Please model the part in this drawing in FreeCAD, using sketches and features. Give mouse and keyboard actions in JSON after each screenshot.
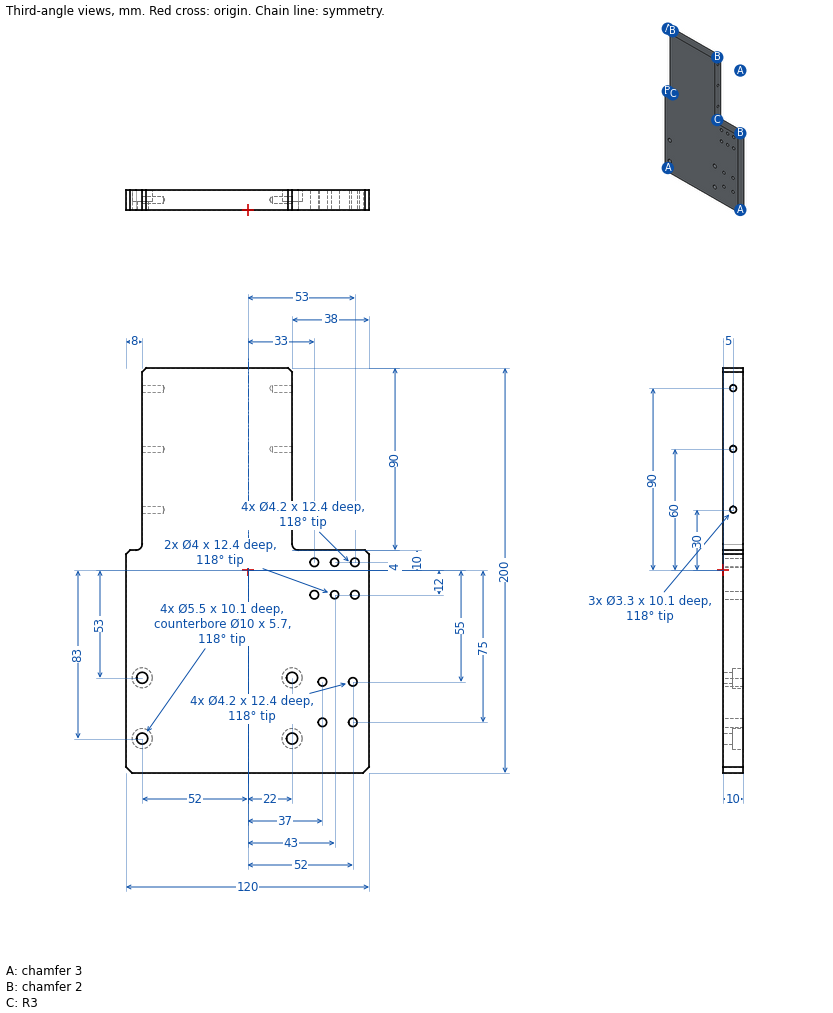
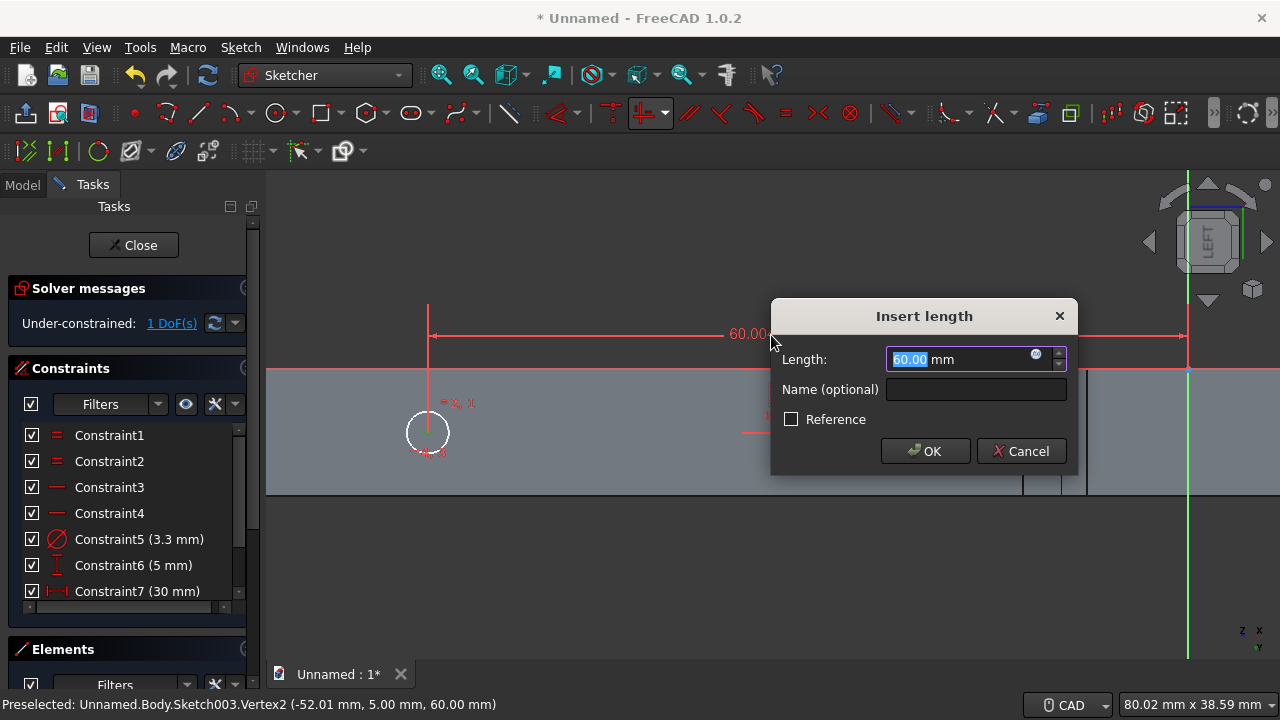
{"action": "type", "text": "60"}
{"action": "key", "text": "Return"}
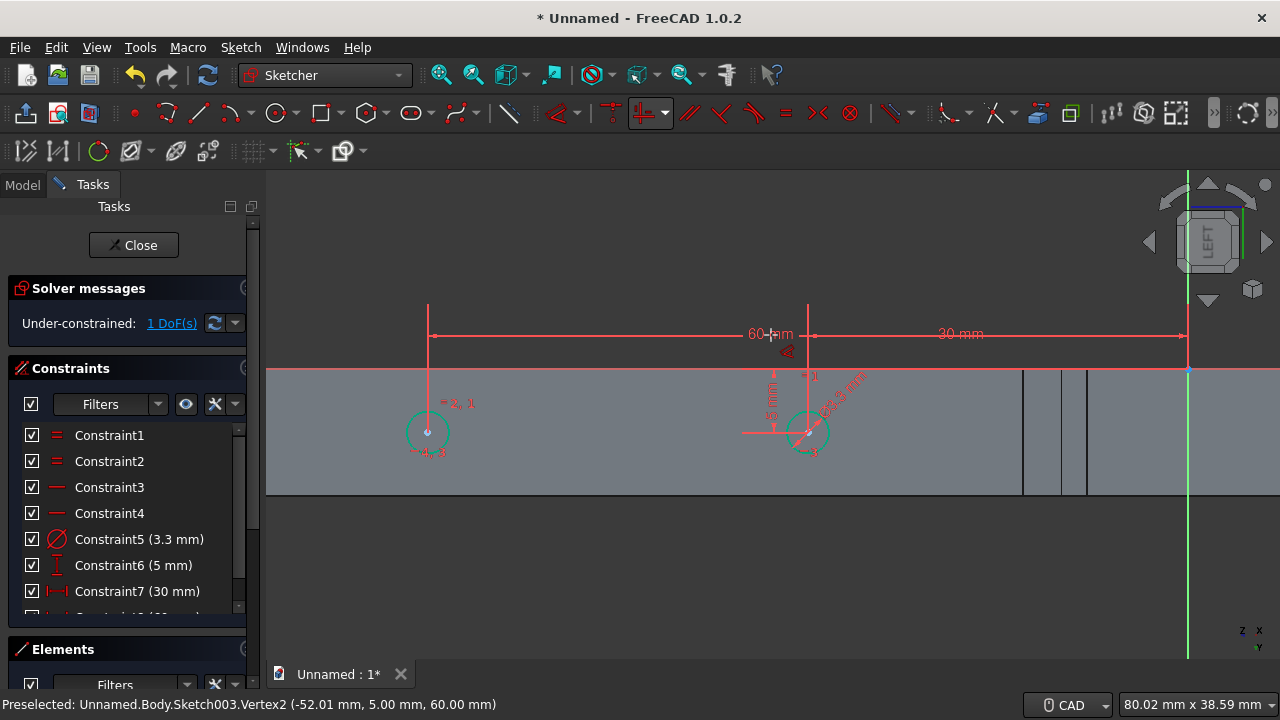
{"action": "scroll", "coordinate": [823, 418], "scroll_direction": "down", "scroll_amount": 3}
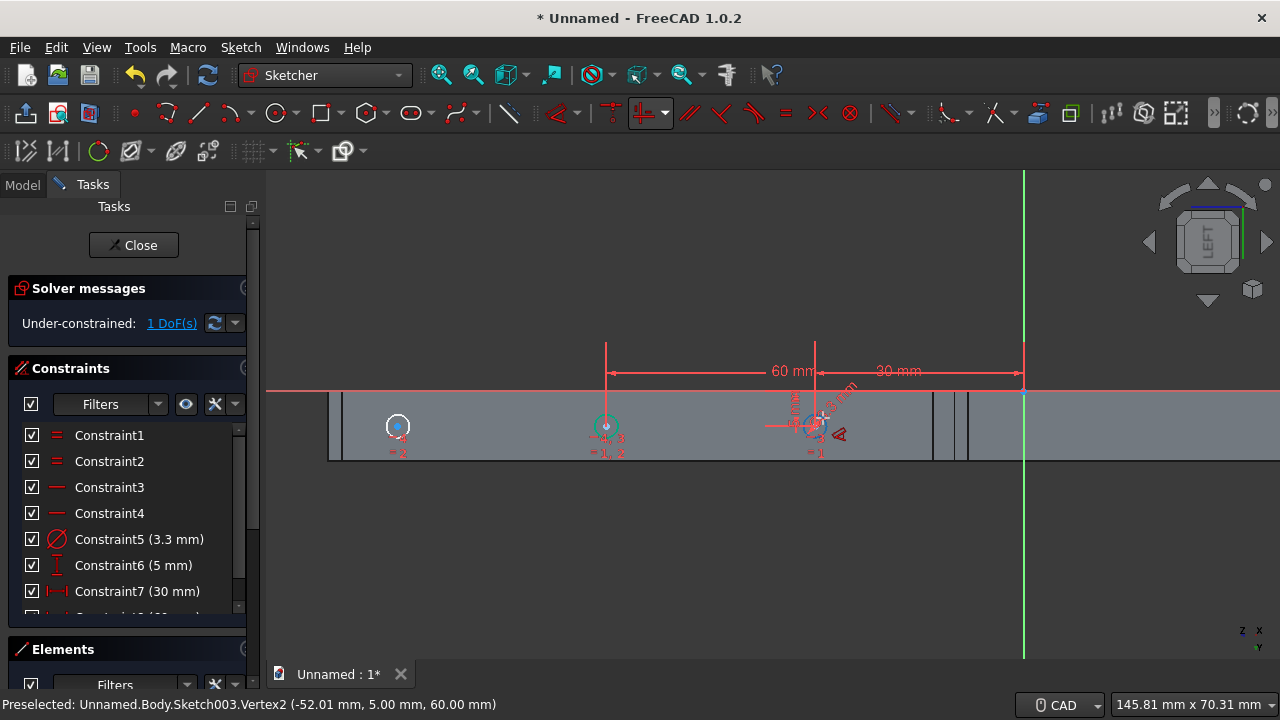
{"action": "left_click", "coordinate": [398, 426]}
{"action": "left_click", "coordinate": [711, 357]}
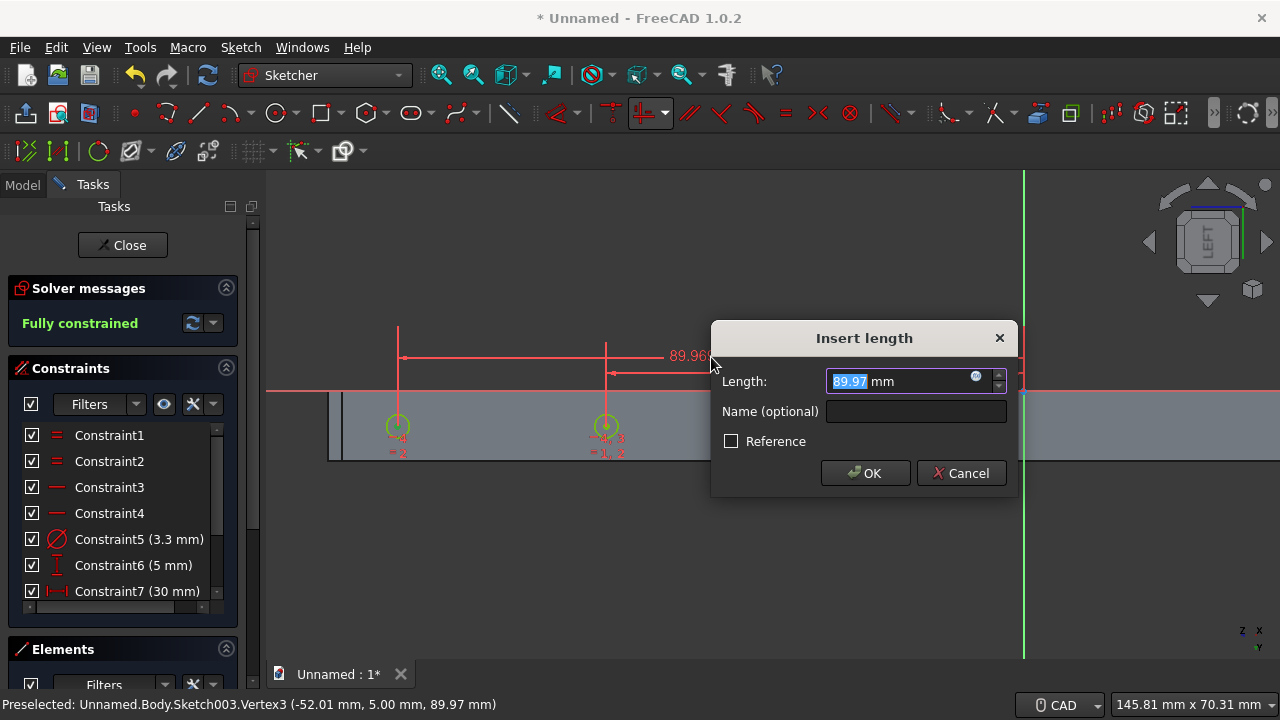
{"action": "type", "text": "90"}
{"action": "key", "text": "Return"}
{"action": "key", "text": "Escape"}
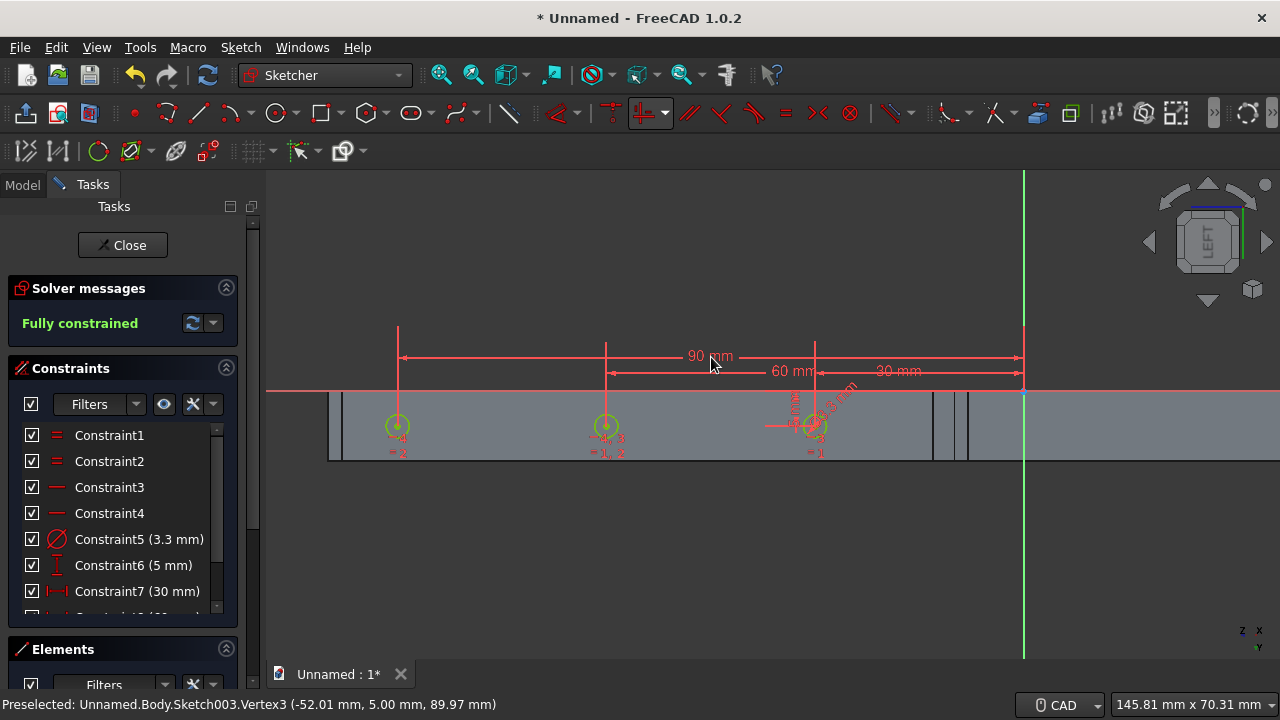
{"action": "left_click", "coordinate": [123, 245]}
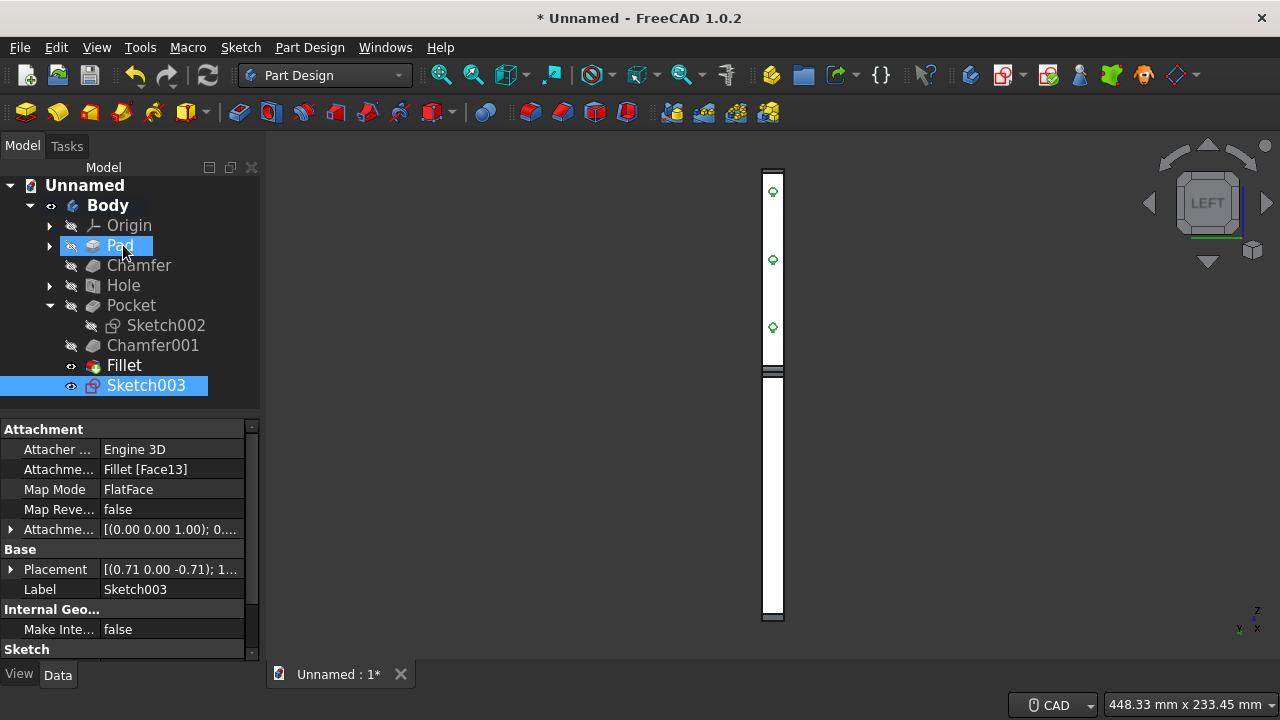
{"action": "left_click", "coordinate": [272, 112]}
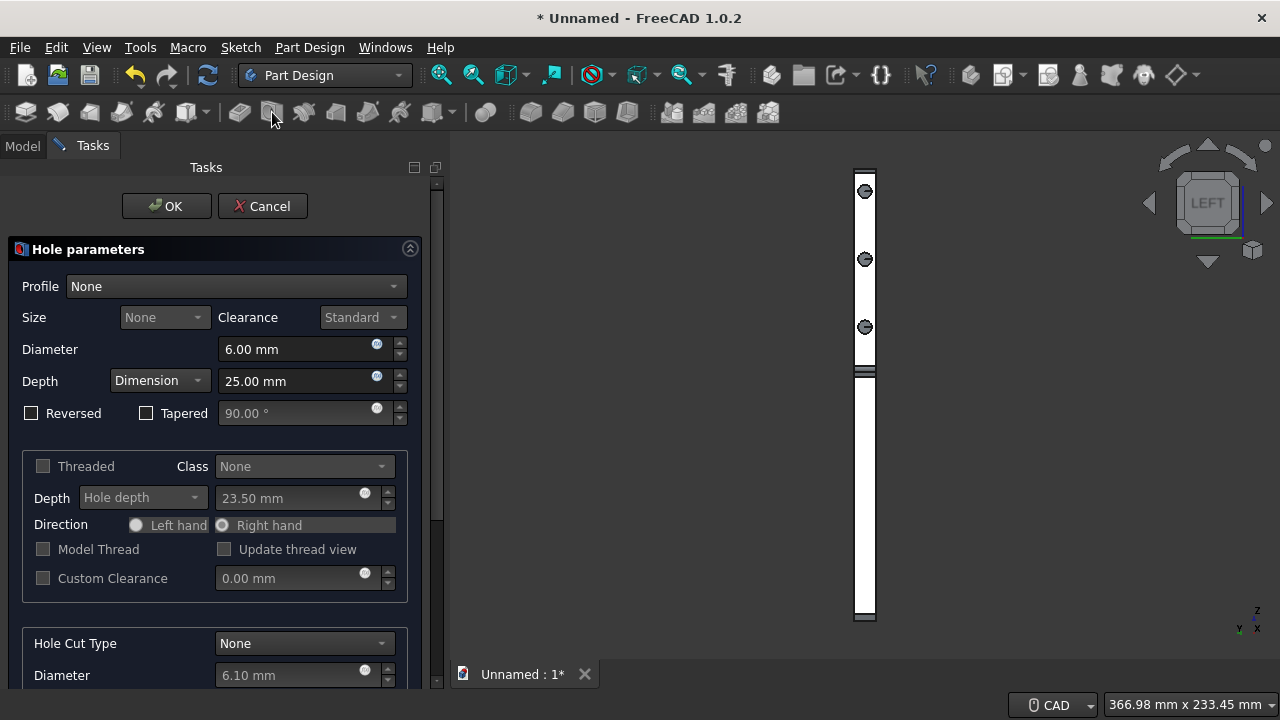
{"action": "triple_click", "coordinate": [305, 349]}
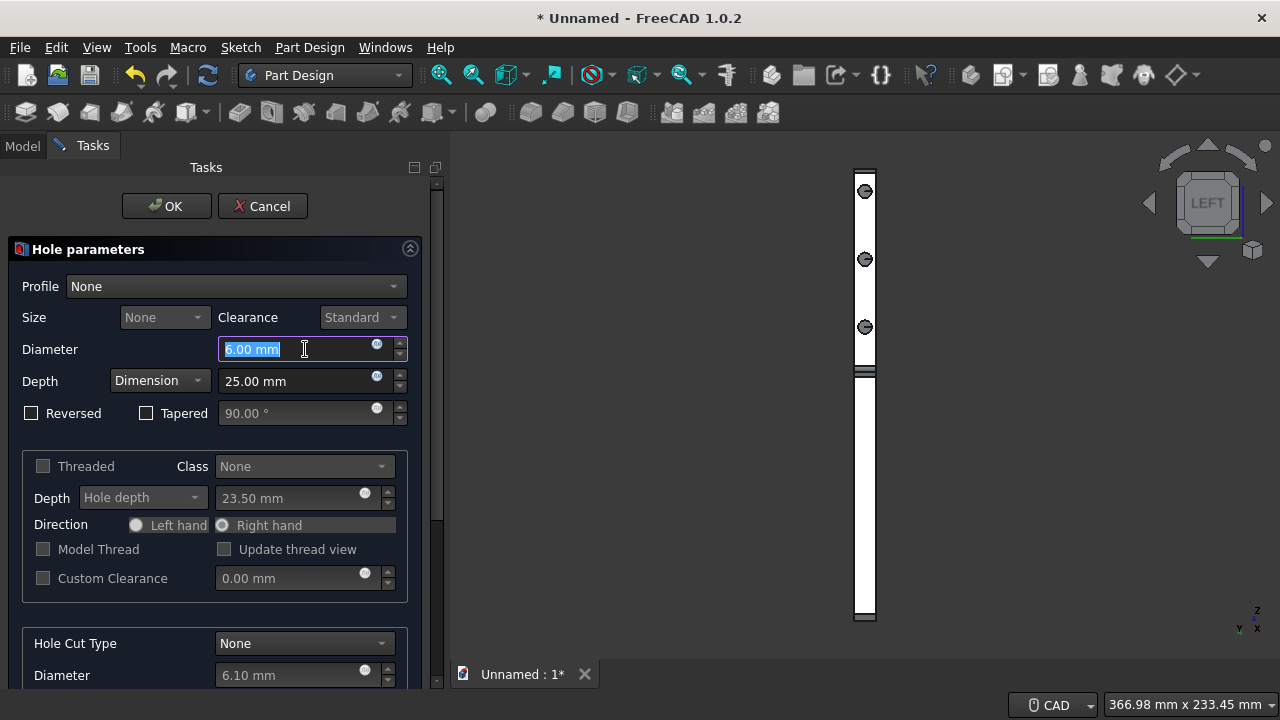
{"action": "type", "text": "3.3"}
{"action": "key", "text": "Tab"}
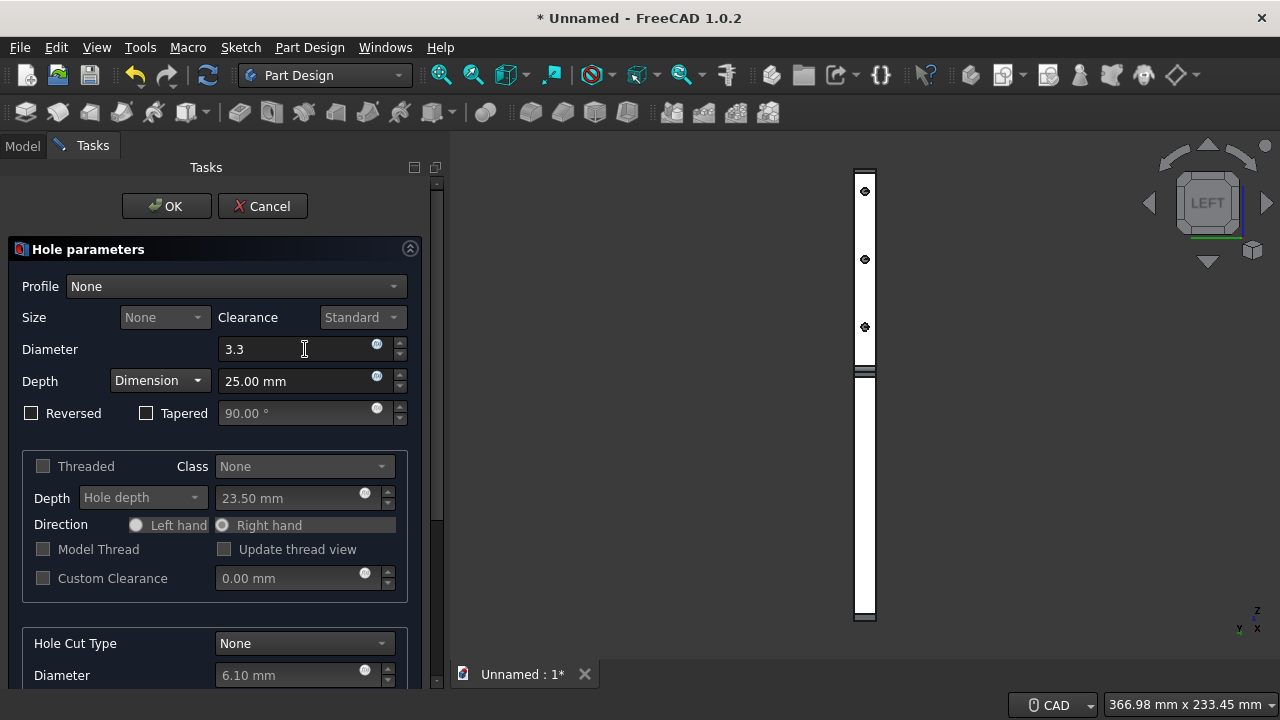
{"action": "triple_click", "coordinate": [305, 381]}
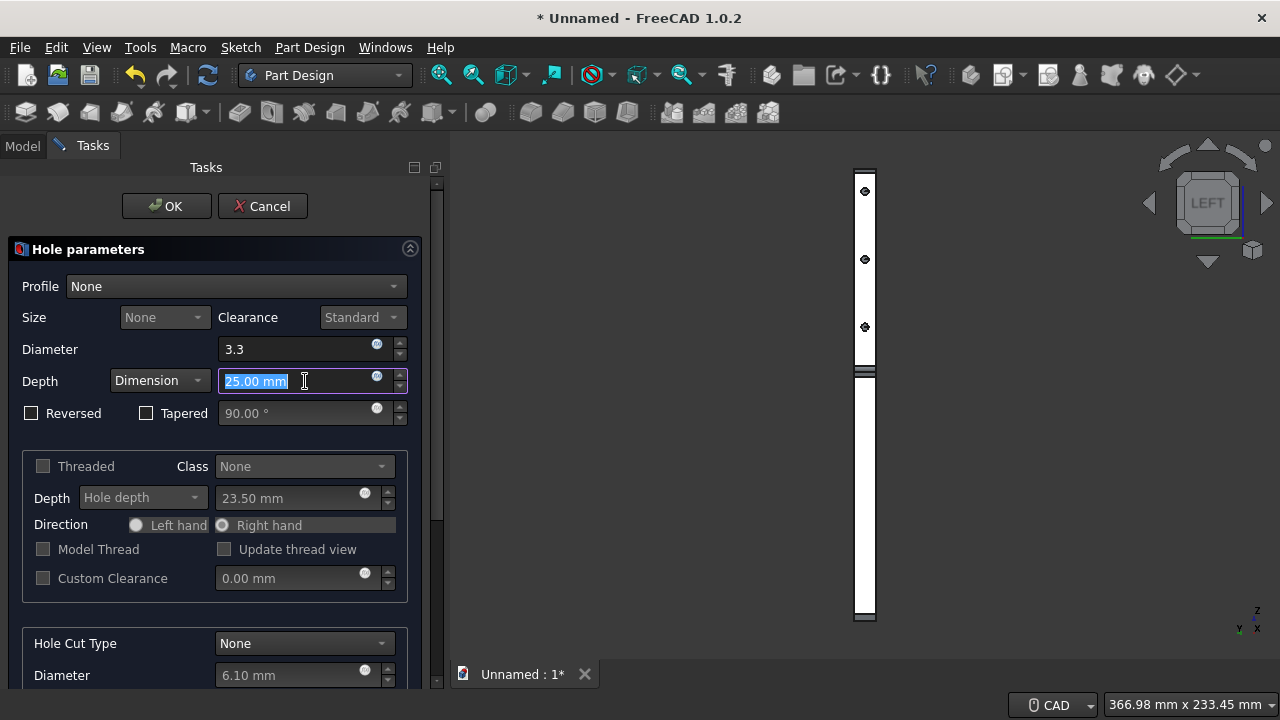
{"action": "type", "text": "10.1"}
{"action": "key", "text": "Tab"}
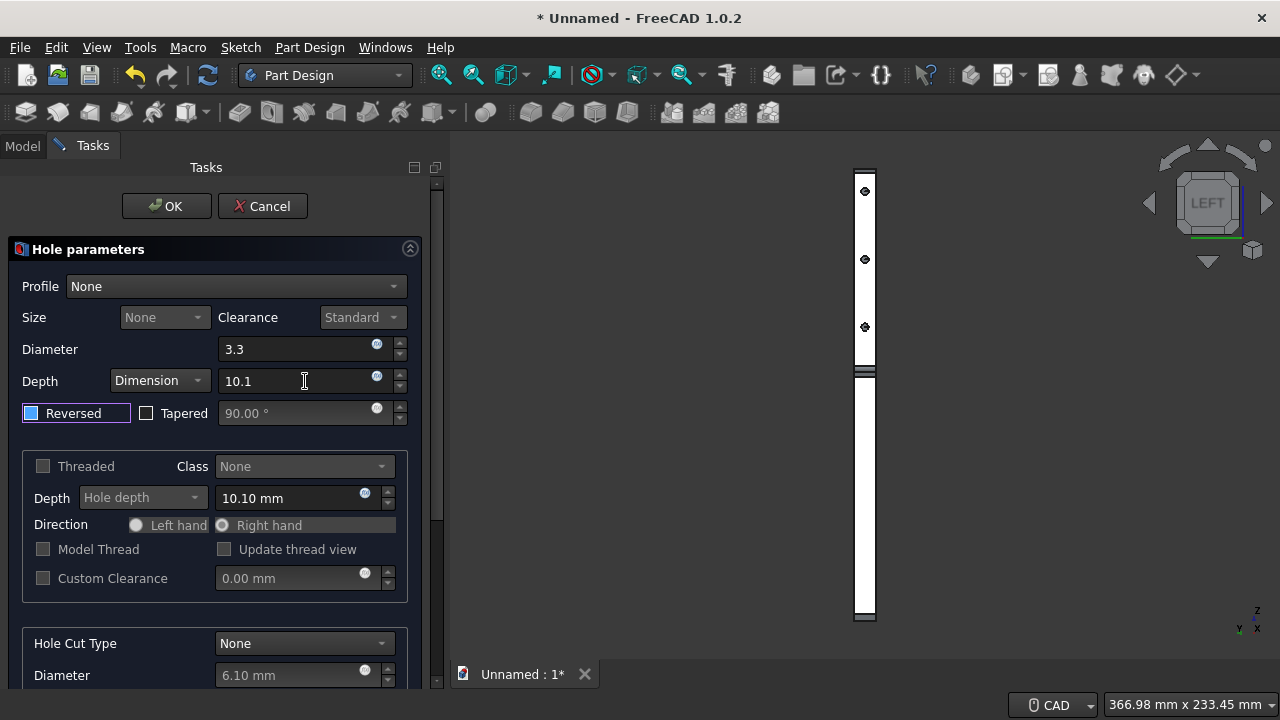
{"action": "left_click", "coordinate": [167, 206]}